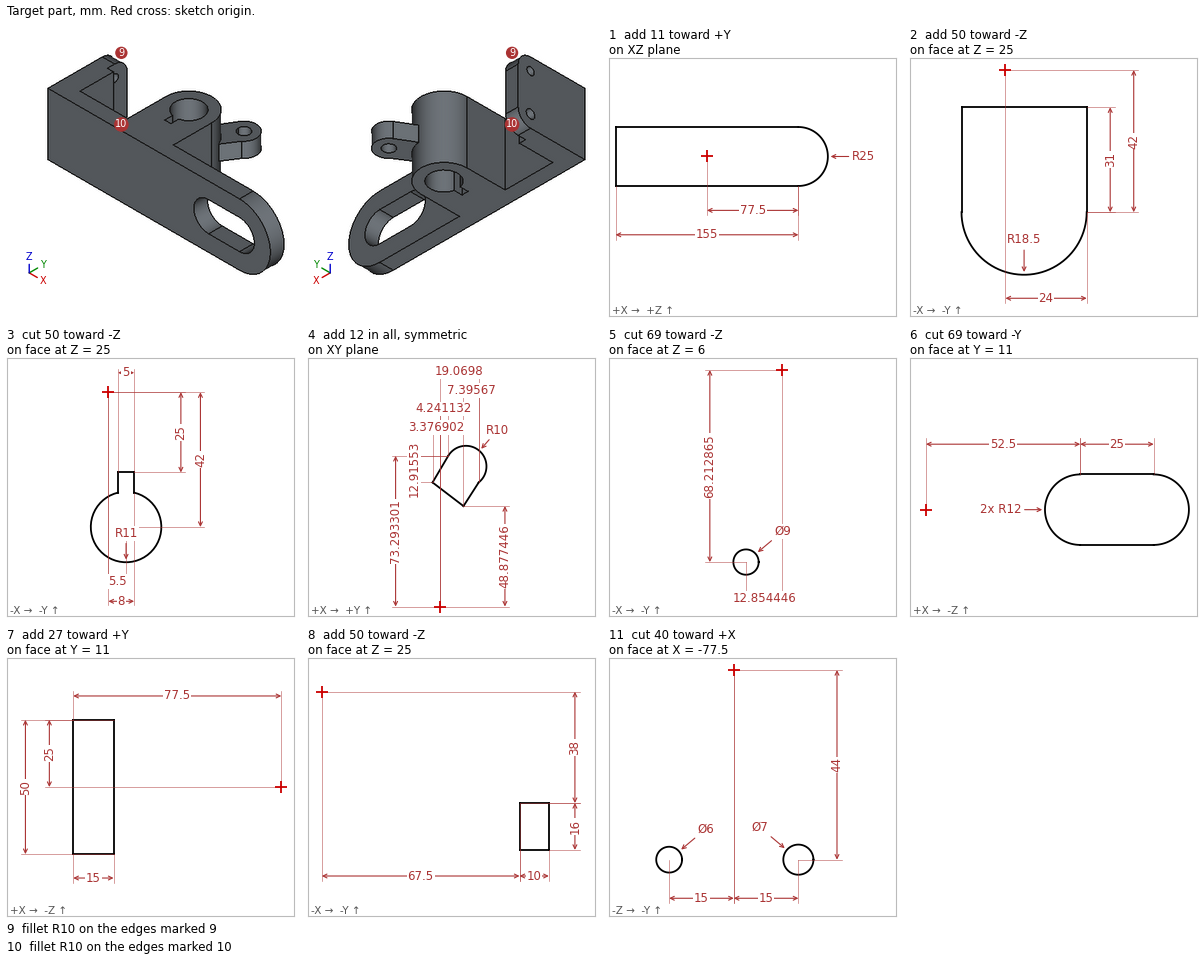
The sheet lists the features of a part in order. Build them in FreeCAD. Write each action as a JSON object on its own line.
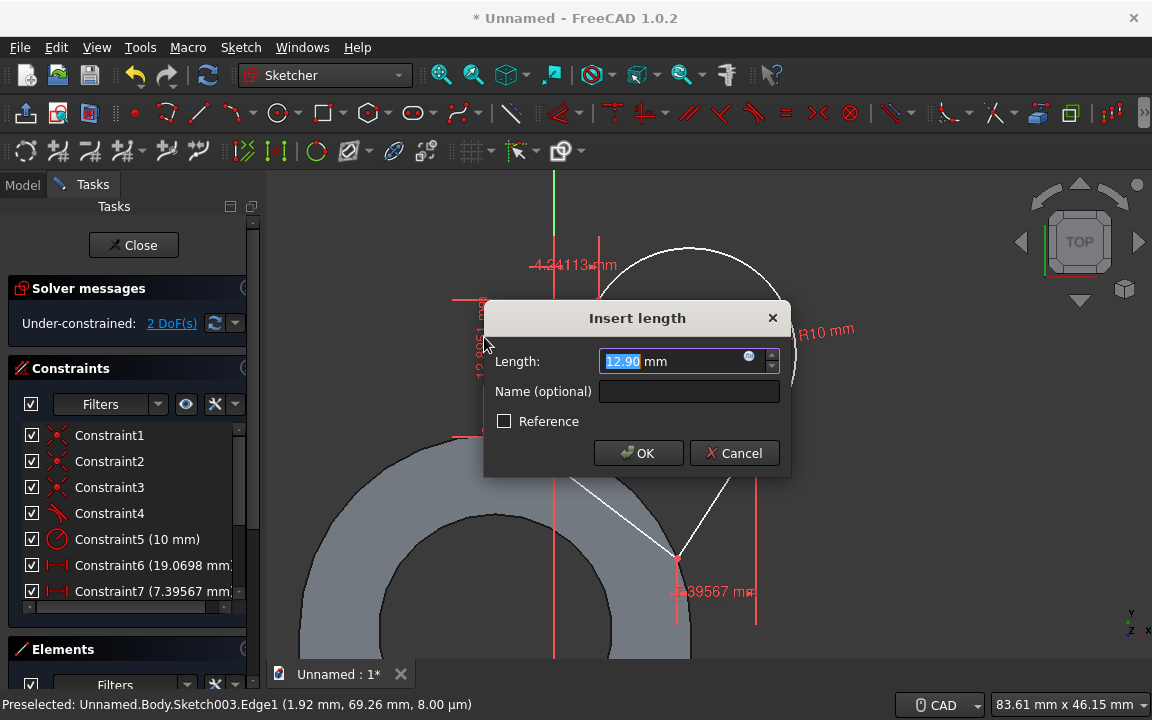
{"action": "type", "text": "12.91553"}
{"action": "key", "text": "Return"}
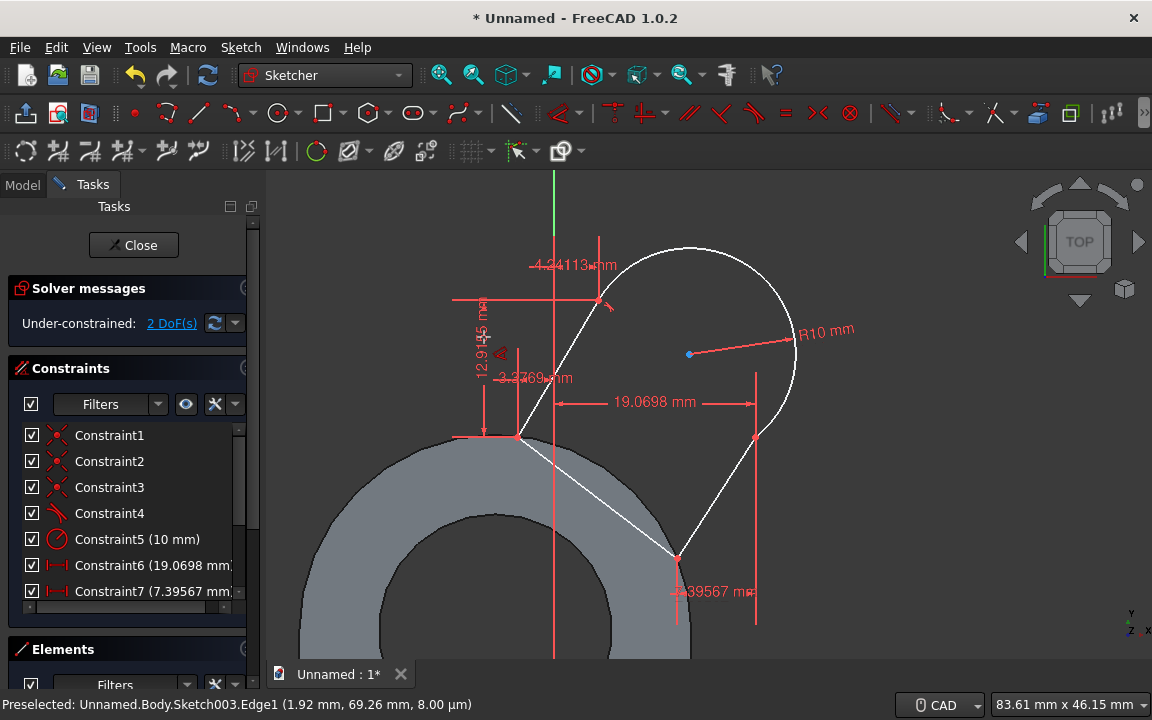
{"action": "left_click", "coordinate": [599, 300]}
{"action": "left_click", "coordinate": [520, 466]}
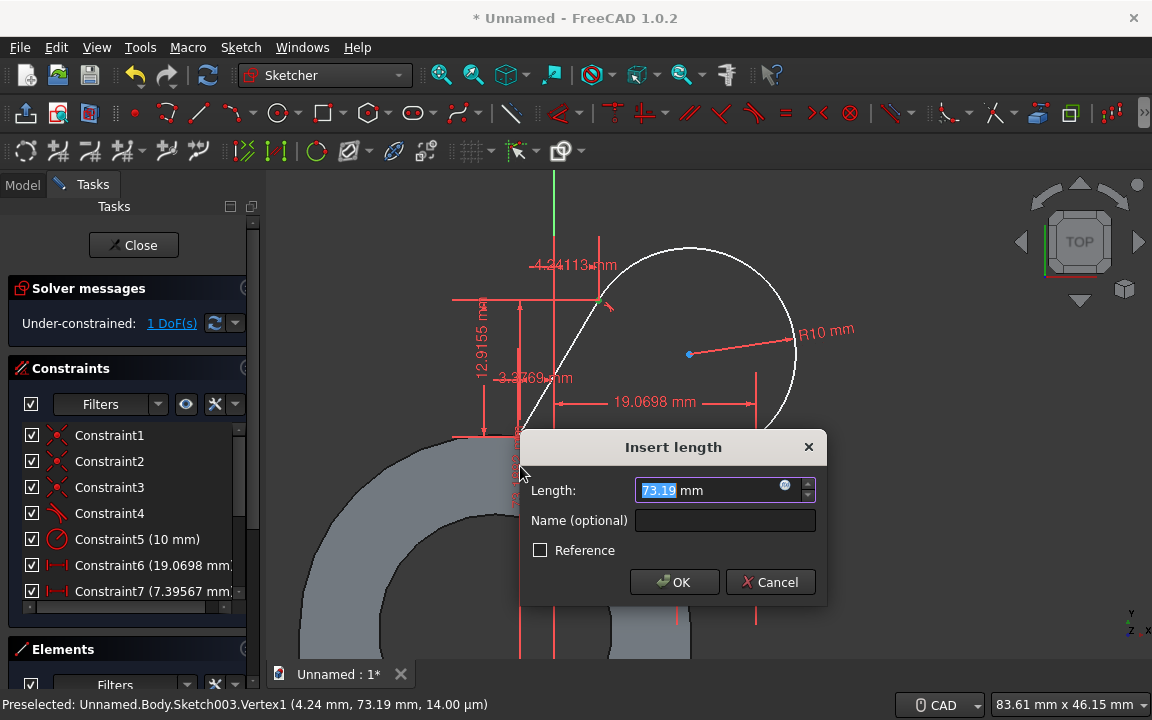
{"action": "type", "text": "73.293301"}
{"action": "key", "text": "Return"}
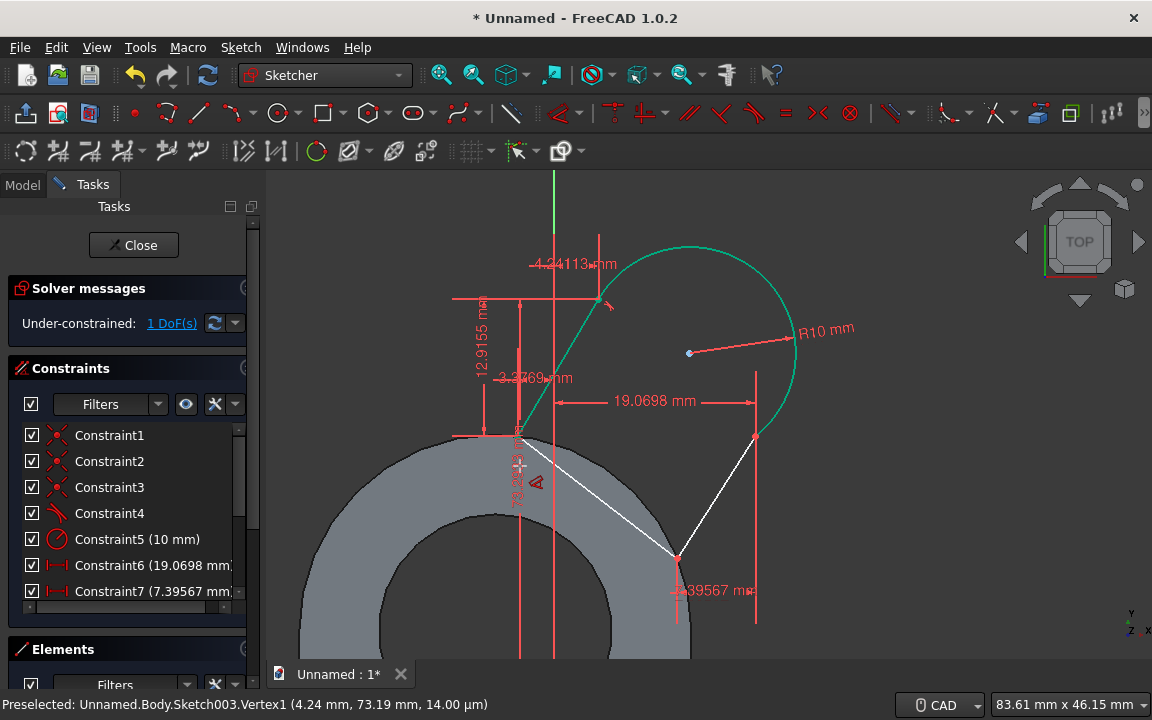
{"action": "left_click", "coordinate": [677, 559]}
{"action": "left_click", "coordinate": [520, 595]}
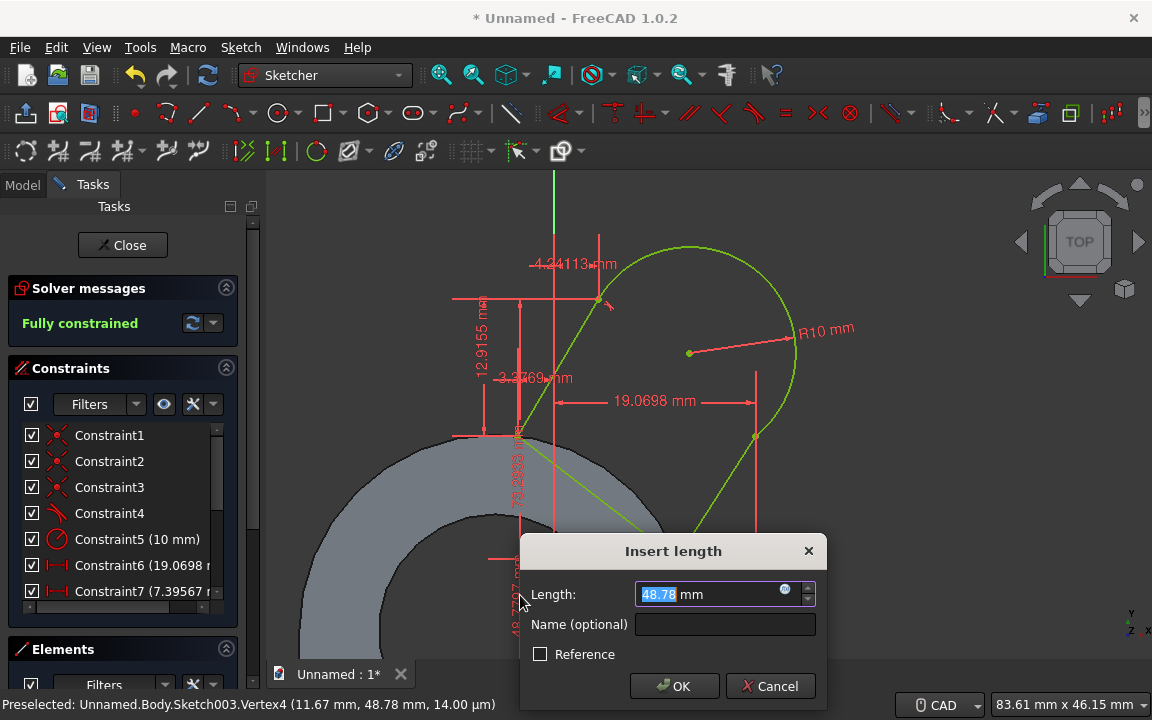
{"action": "type", "text": "48.877446"}
{"action": "key", "text": "Return"}
{"action": "key", "text": "Escape"}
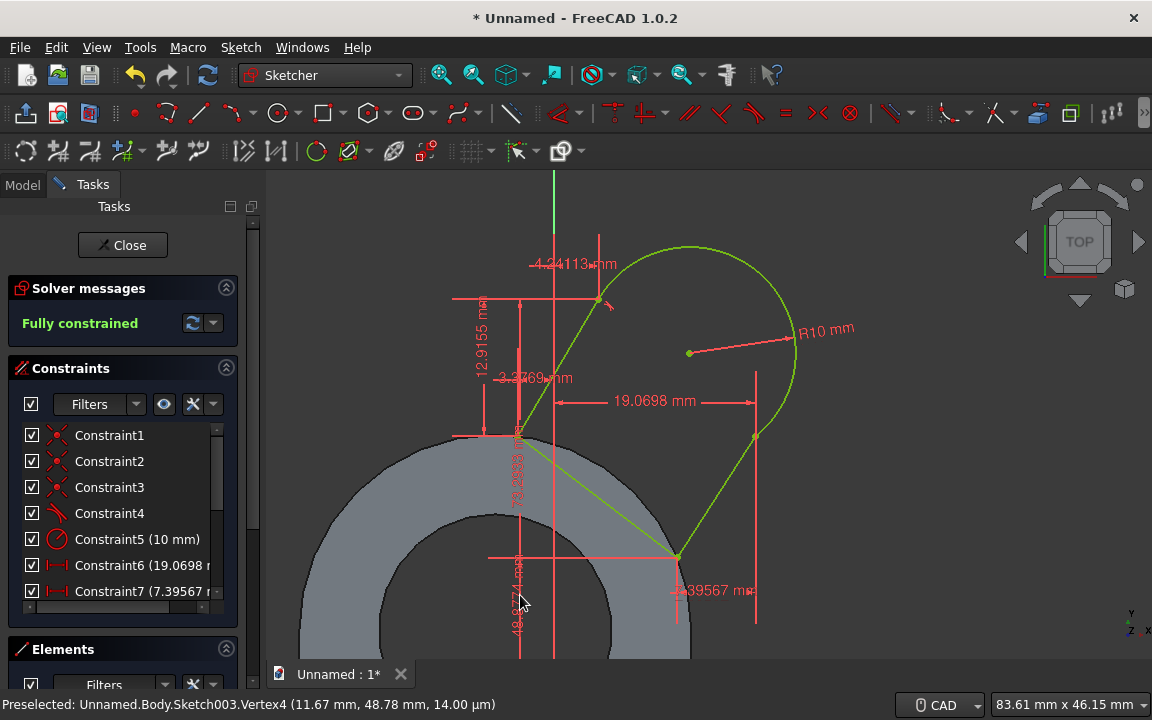
{"action": "left_click", "coordinate": [123, 245]}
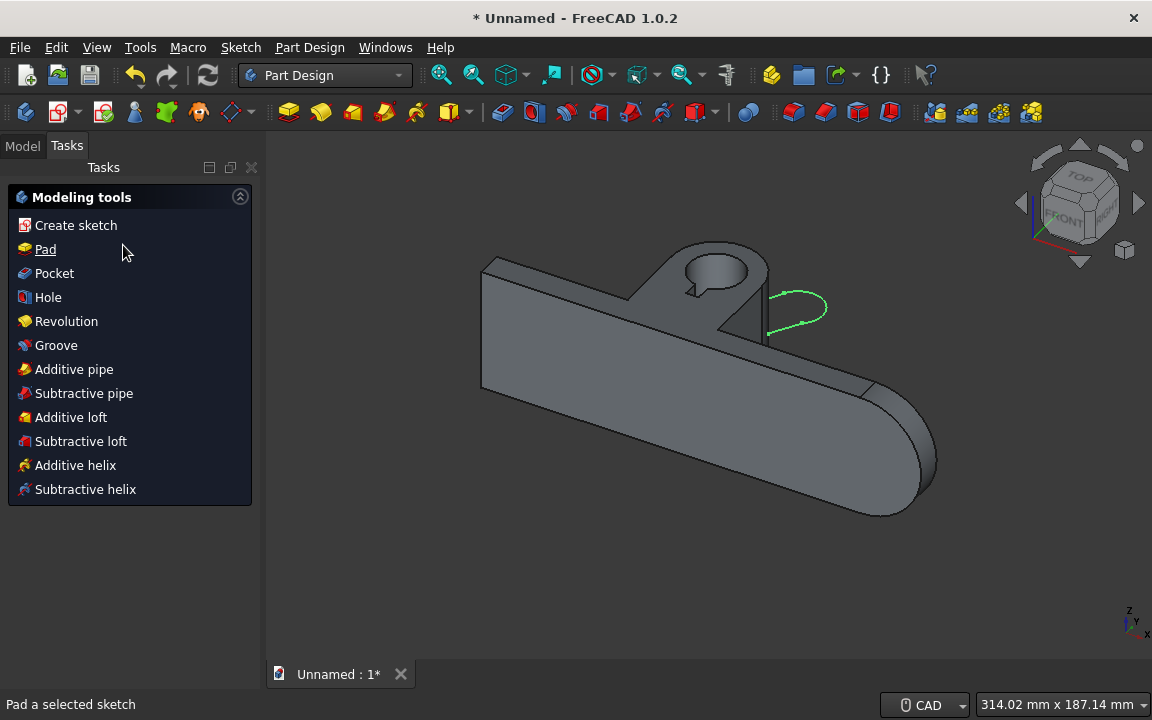
{"action": "left_click", "coordinate": [290, 112]}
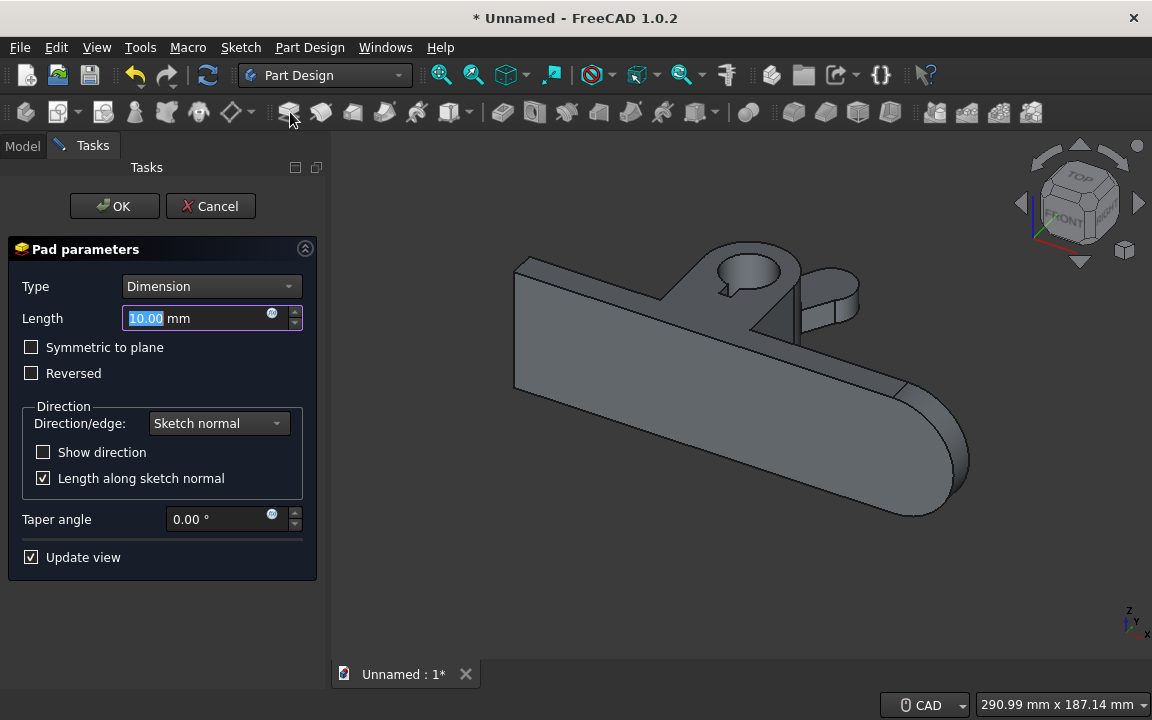
{"action": "type", "text": "12"}
{"action": "key", "text": "Tab"}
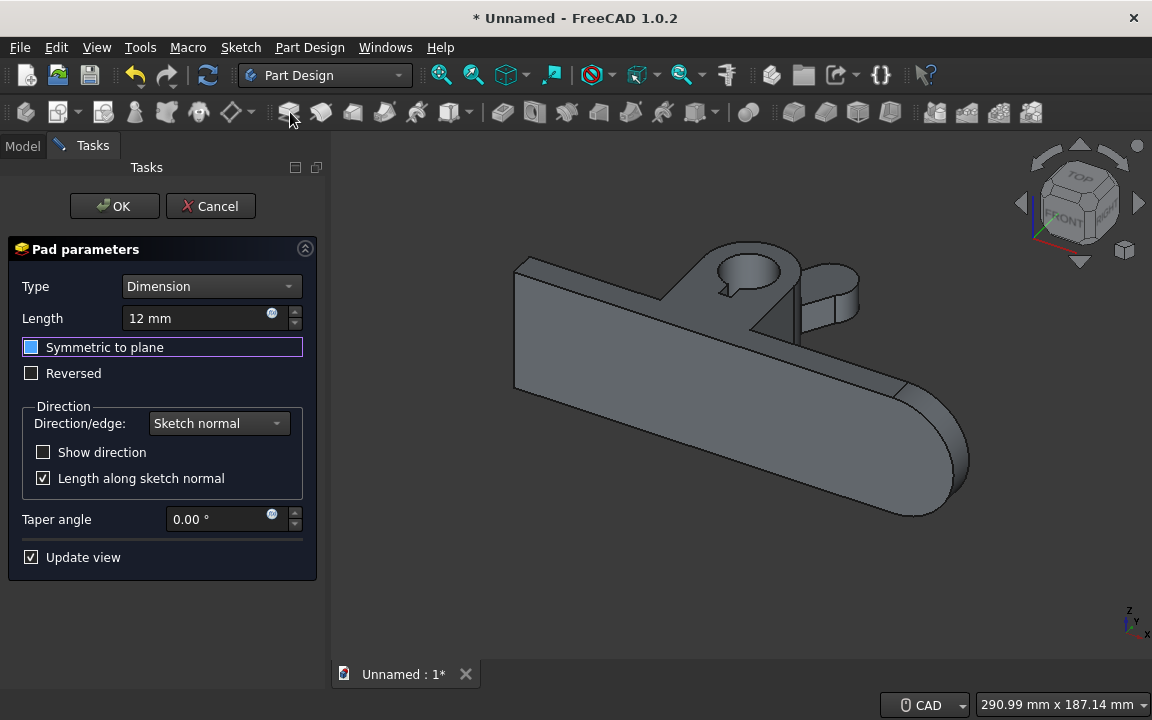
{"action": "left_click", "coordinate": [30, 347]}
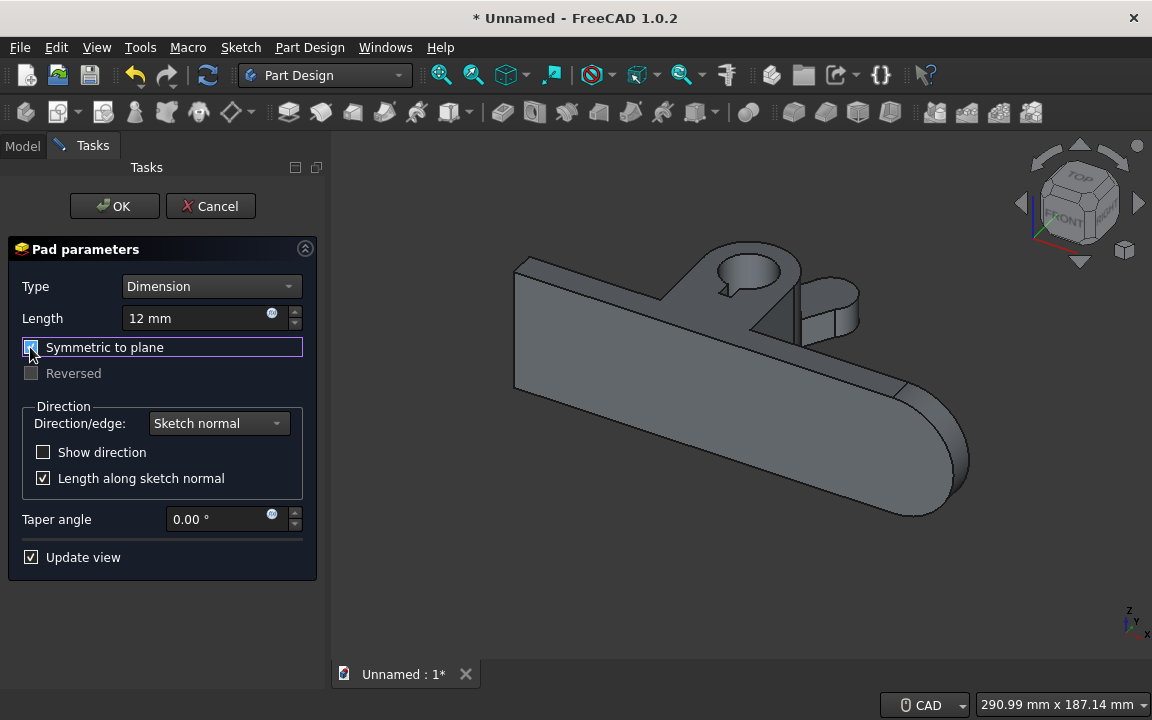
{"action": "left_click", "coordinate": [115, 206]}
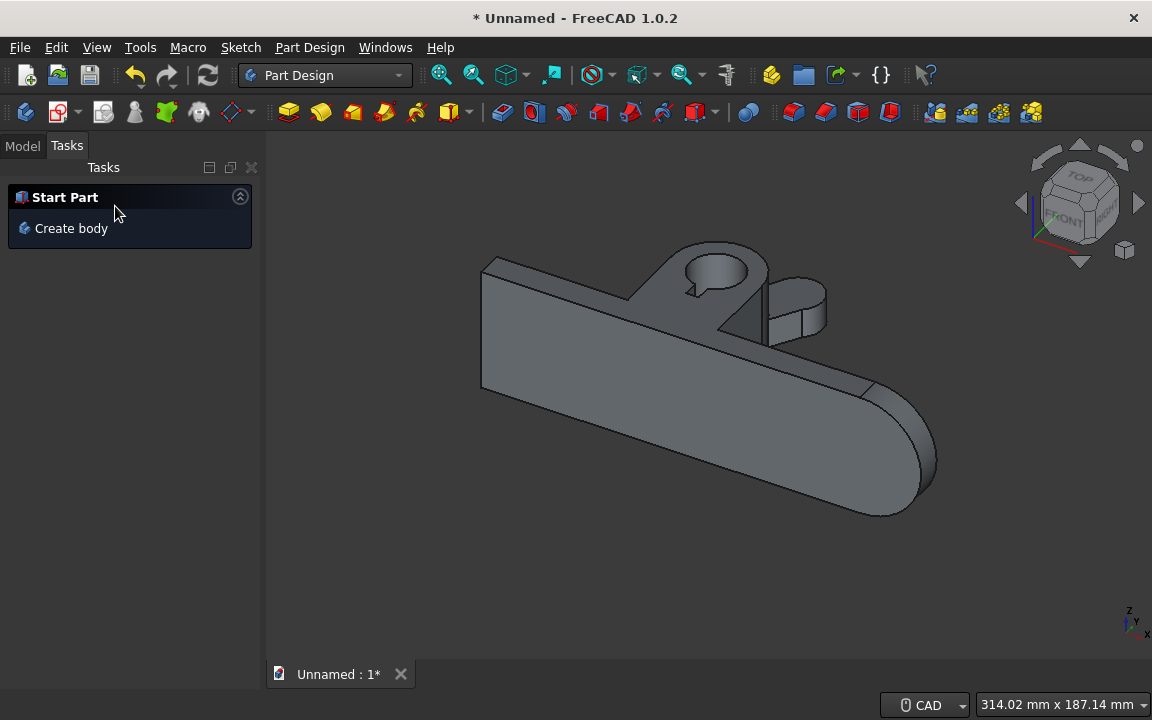
{"action": "left_click", "coordinate": [799, 294]}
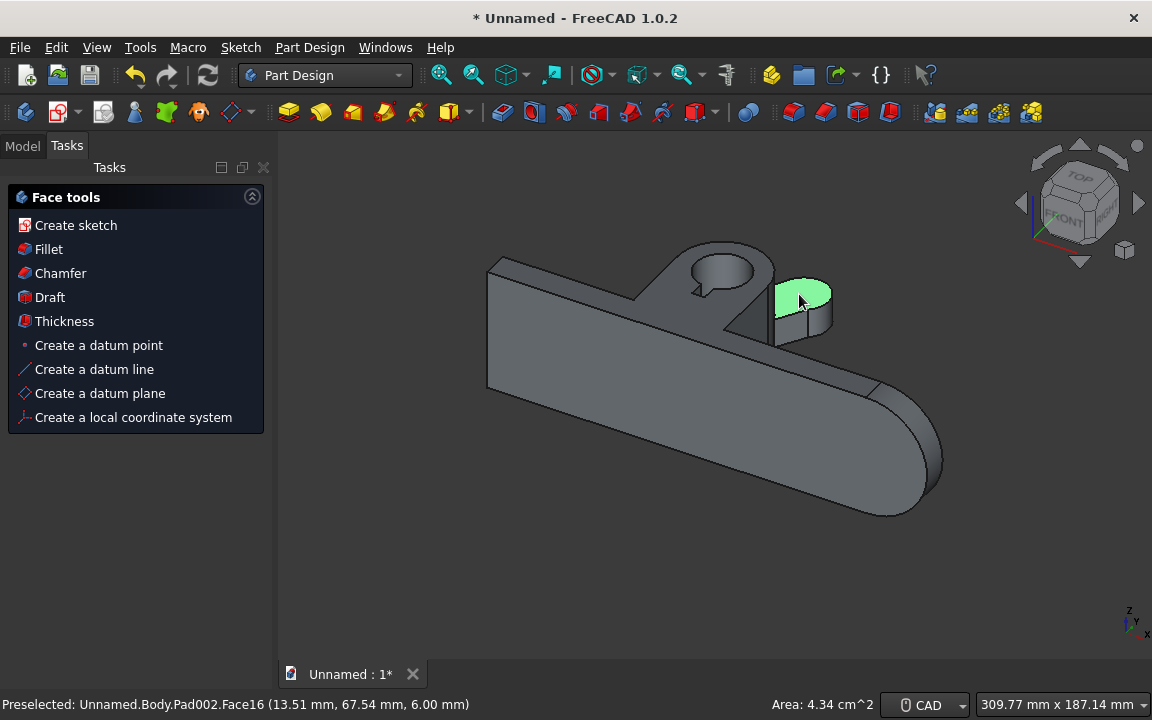
{"action": "left_click", "coordinate": [58, 112]}